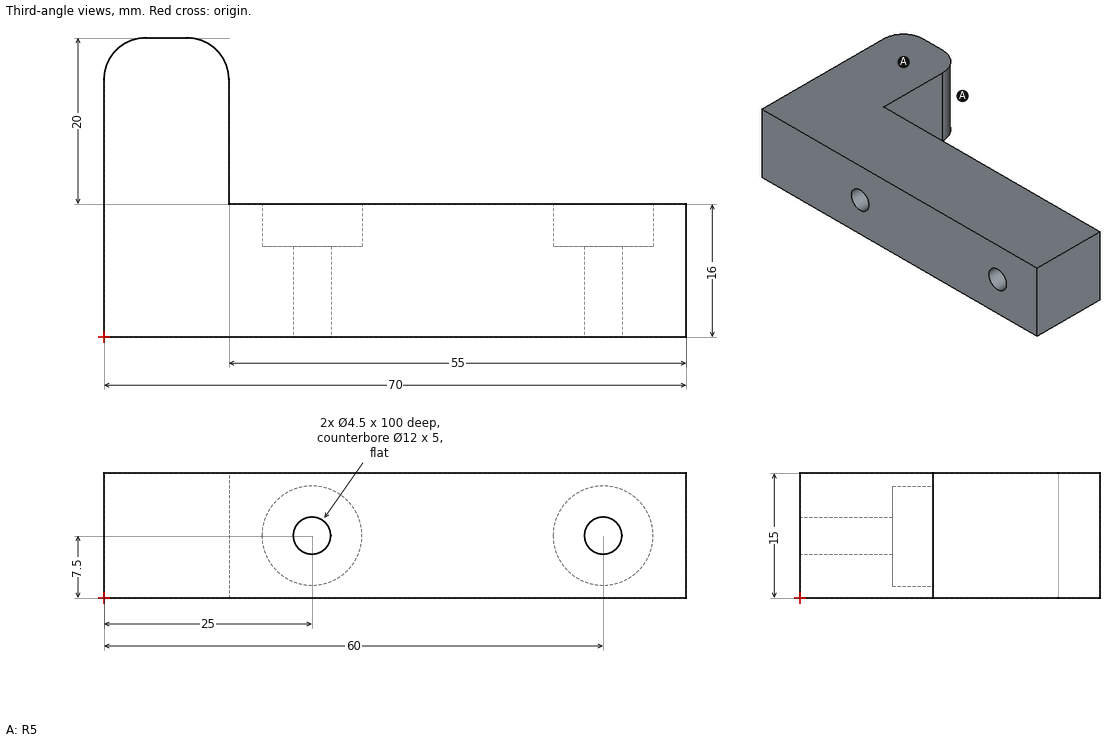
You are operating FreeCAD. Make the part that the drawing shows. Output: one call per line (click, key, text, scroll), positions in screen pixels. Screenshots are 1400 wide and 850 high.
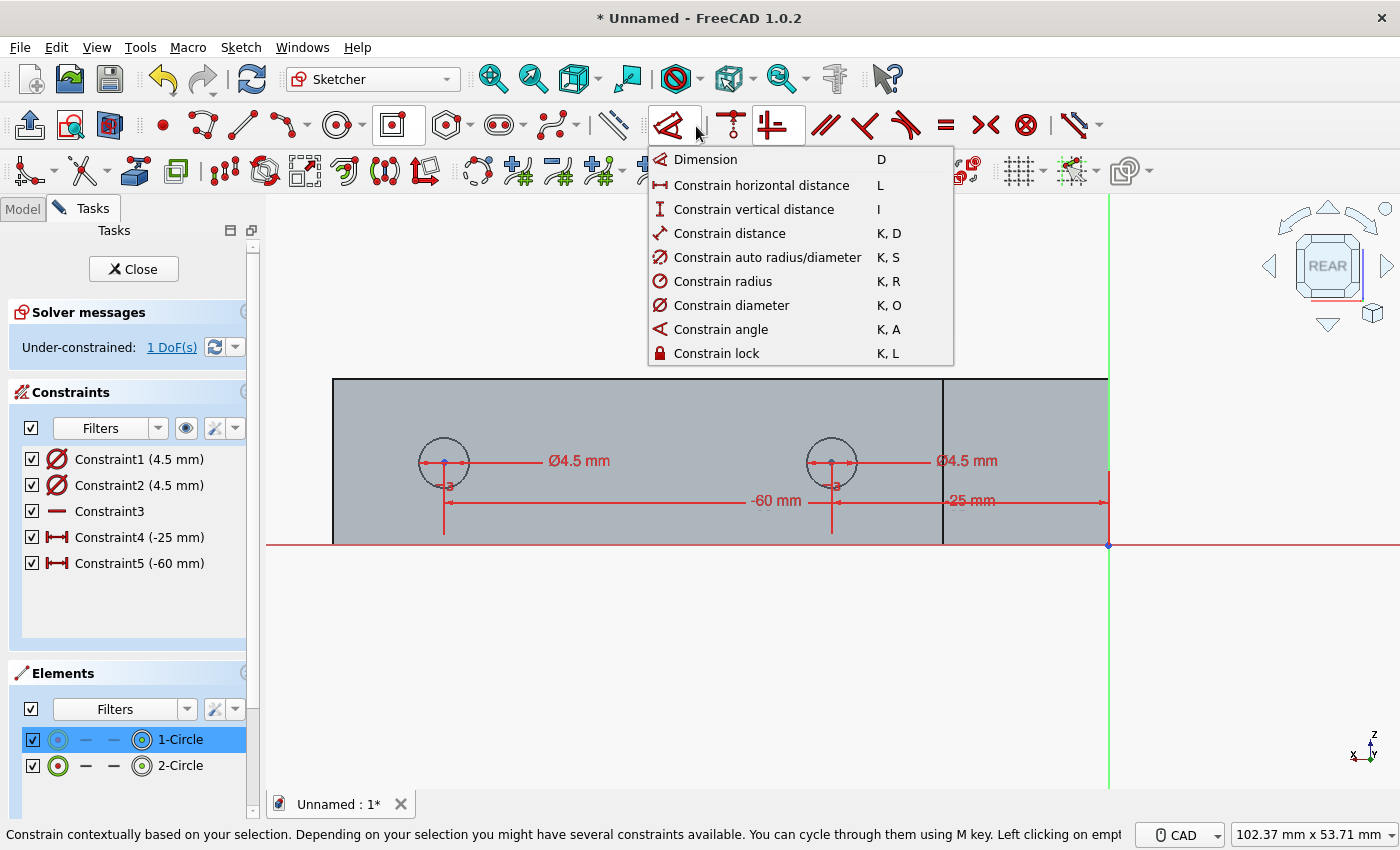
click(801, 209)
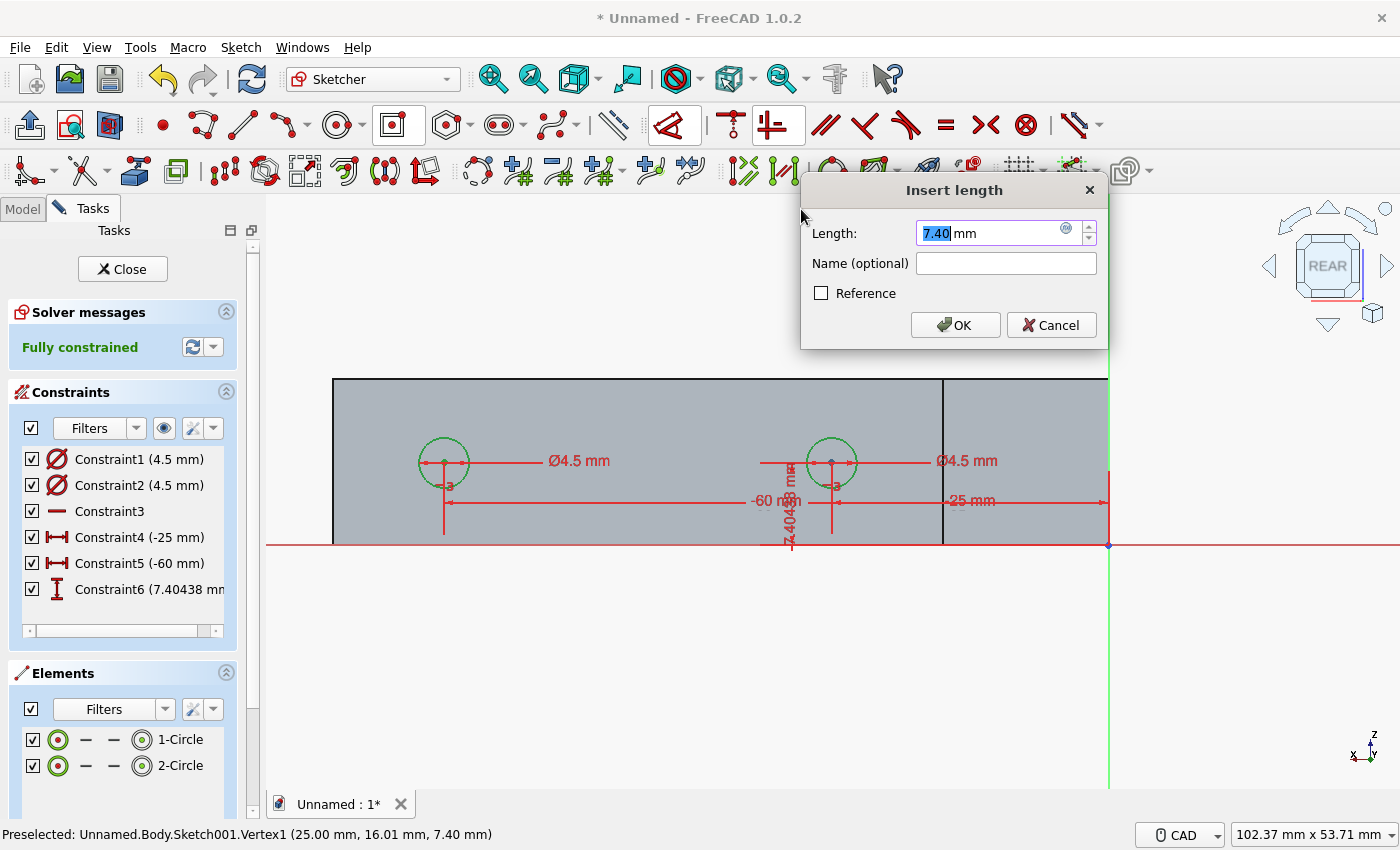
text(7.5)
key(Return)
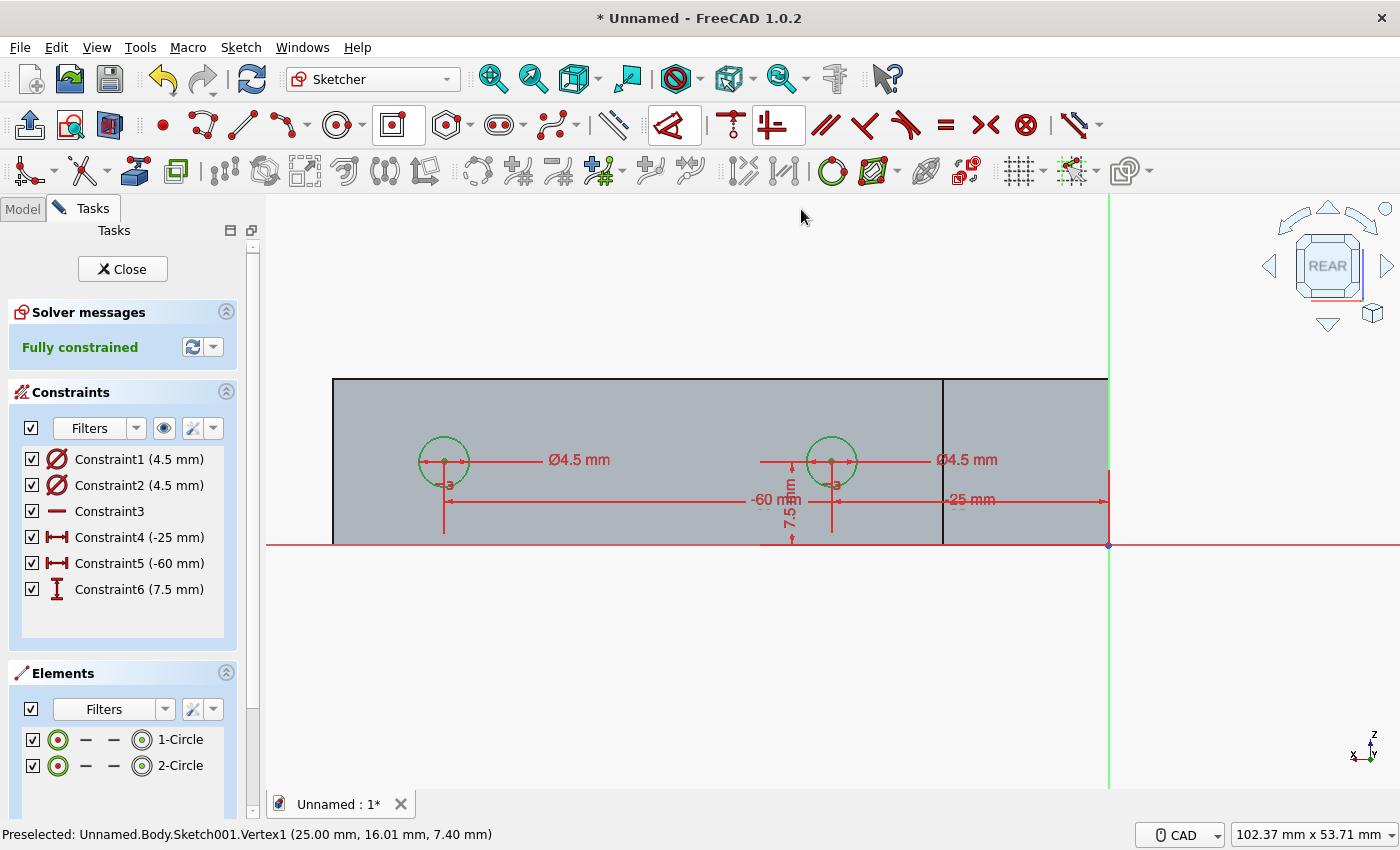
click(123, 269)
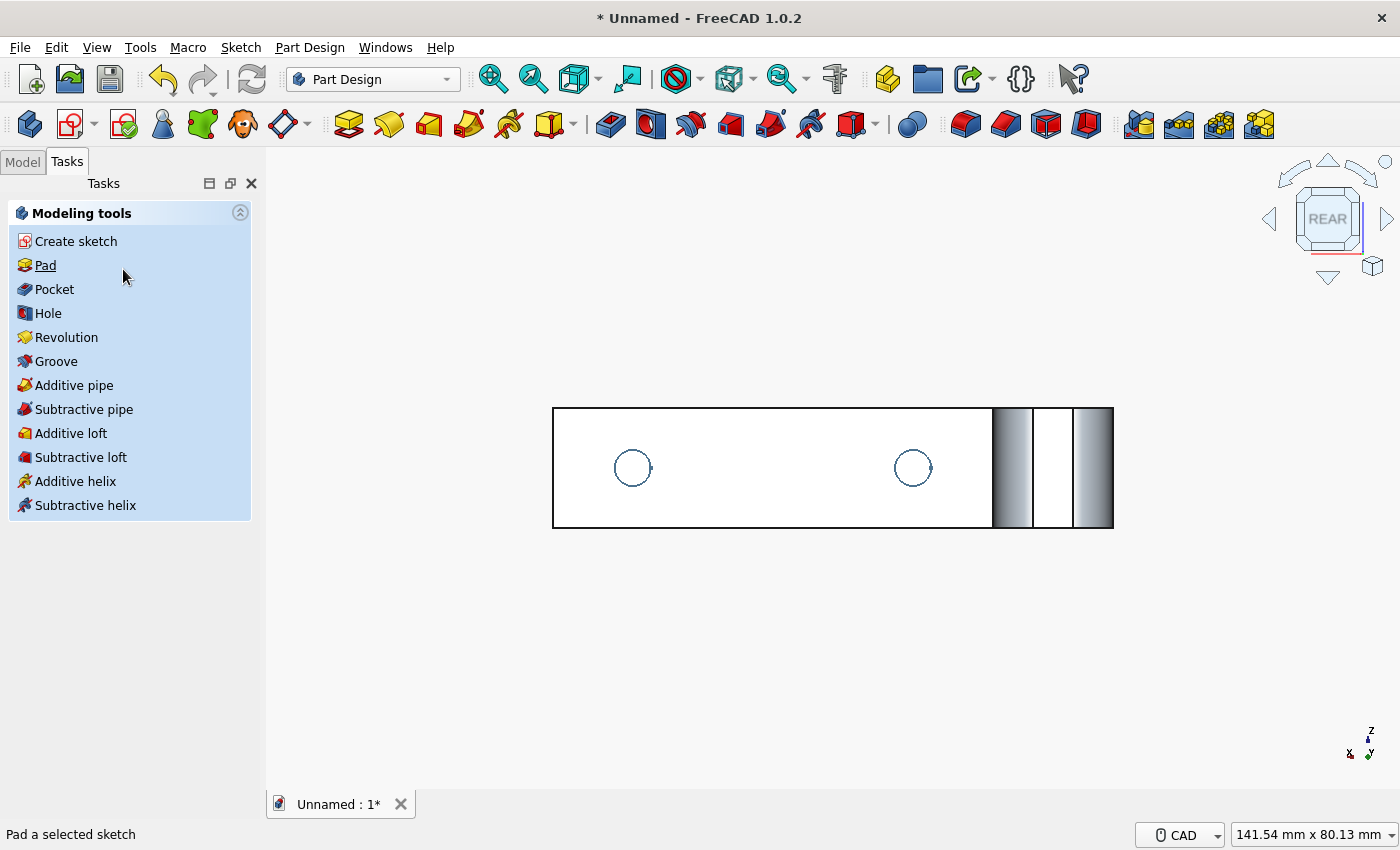
click(652, 124)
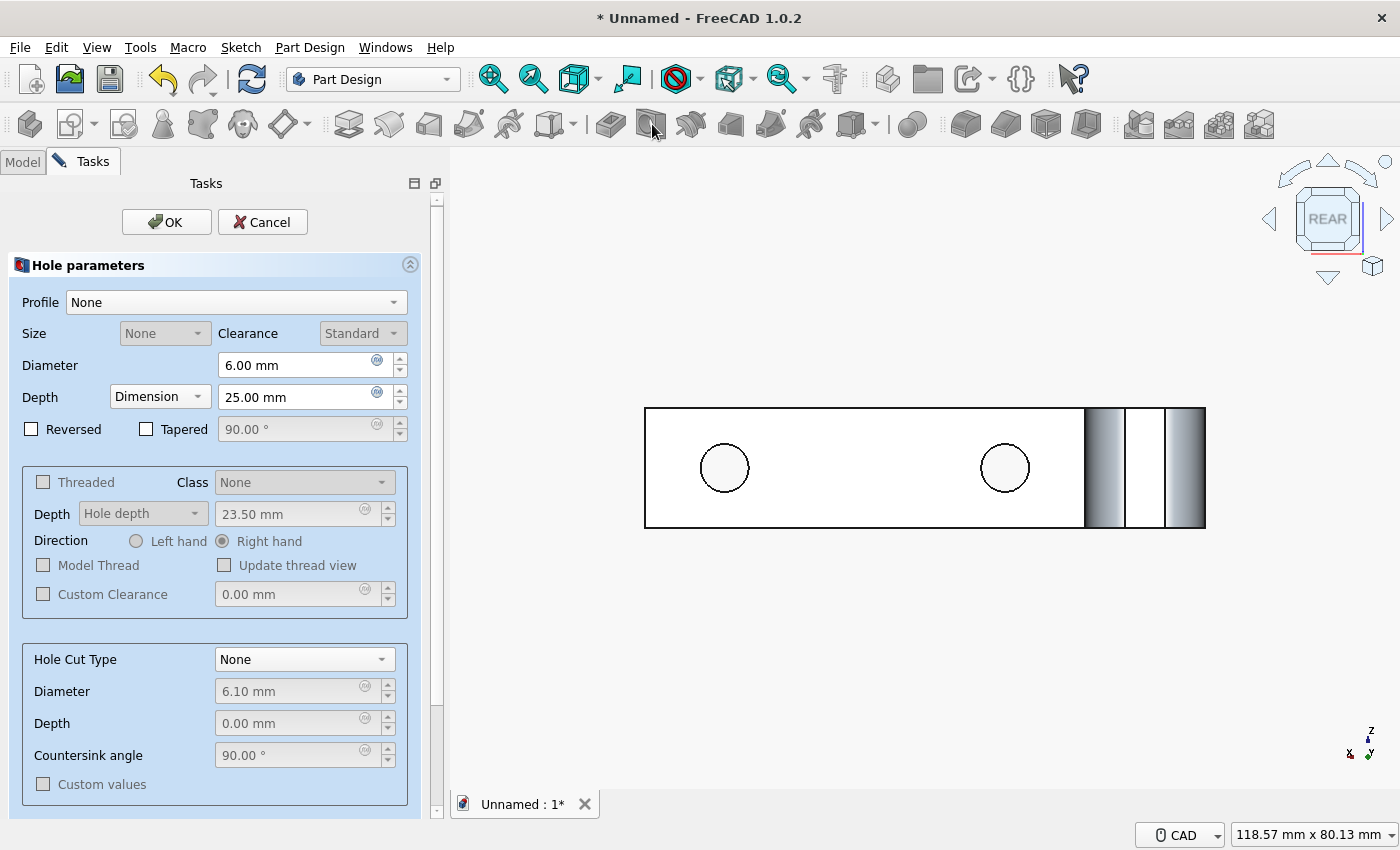
triple_click(305, 365)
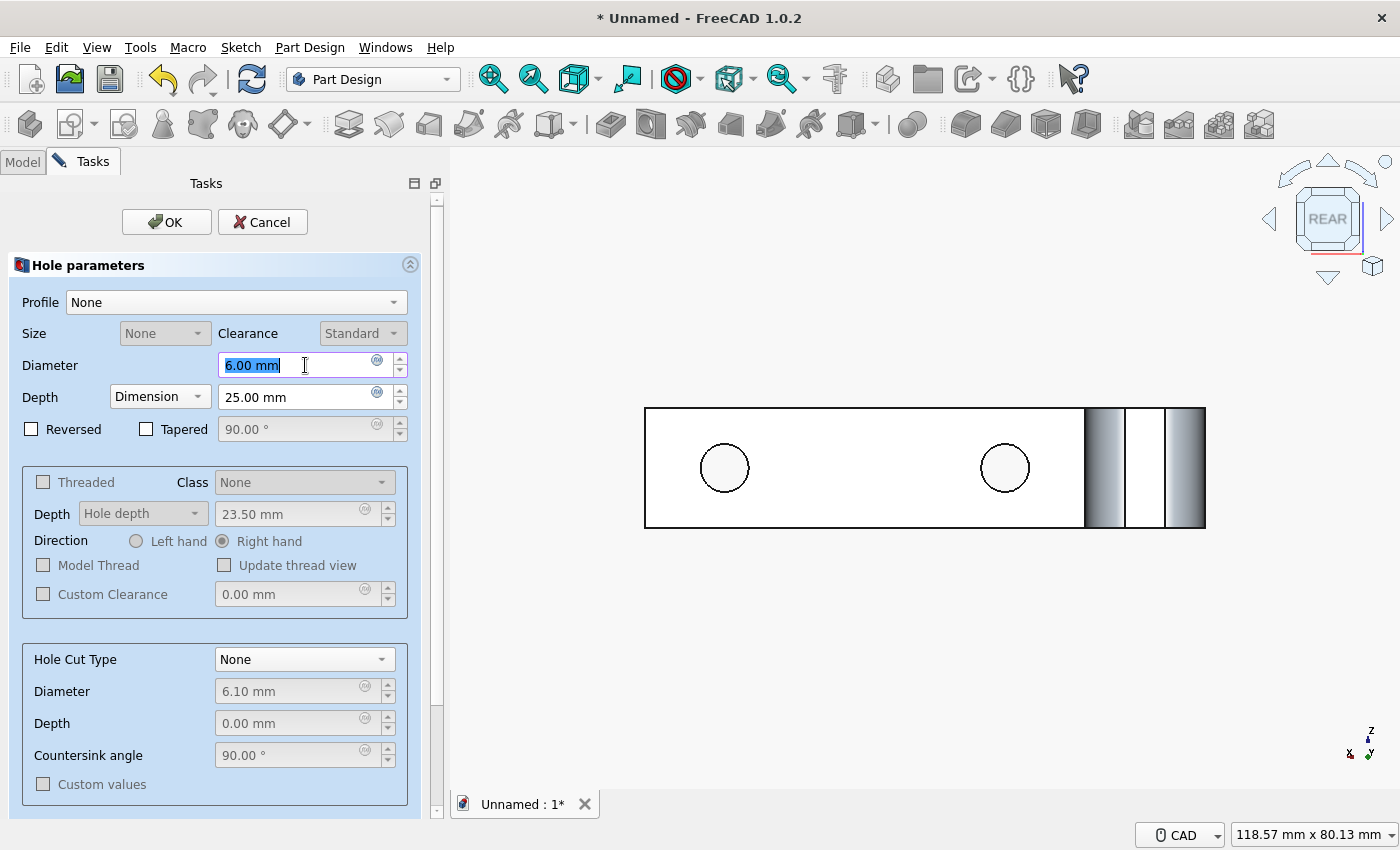
text(4.5)
key(Tab)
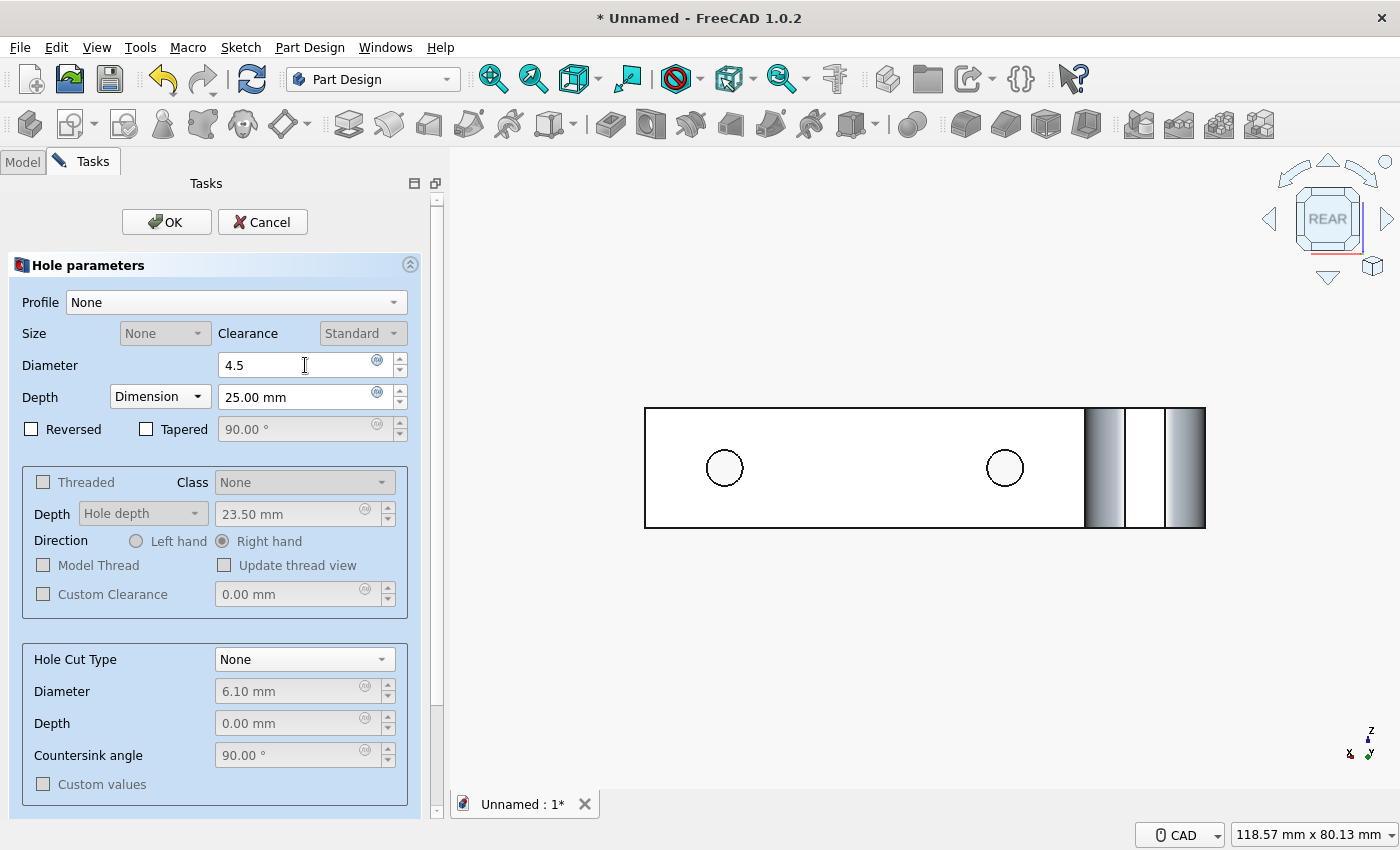
triple_click(305, 397)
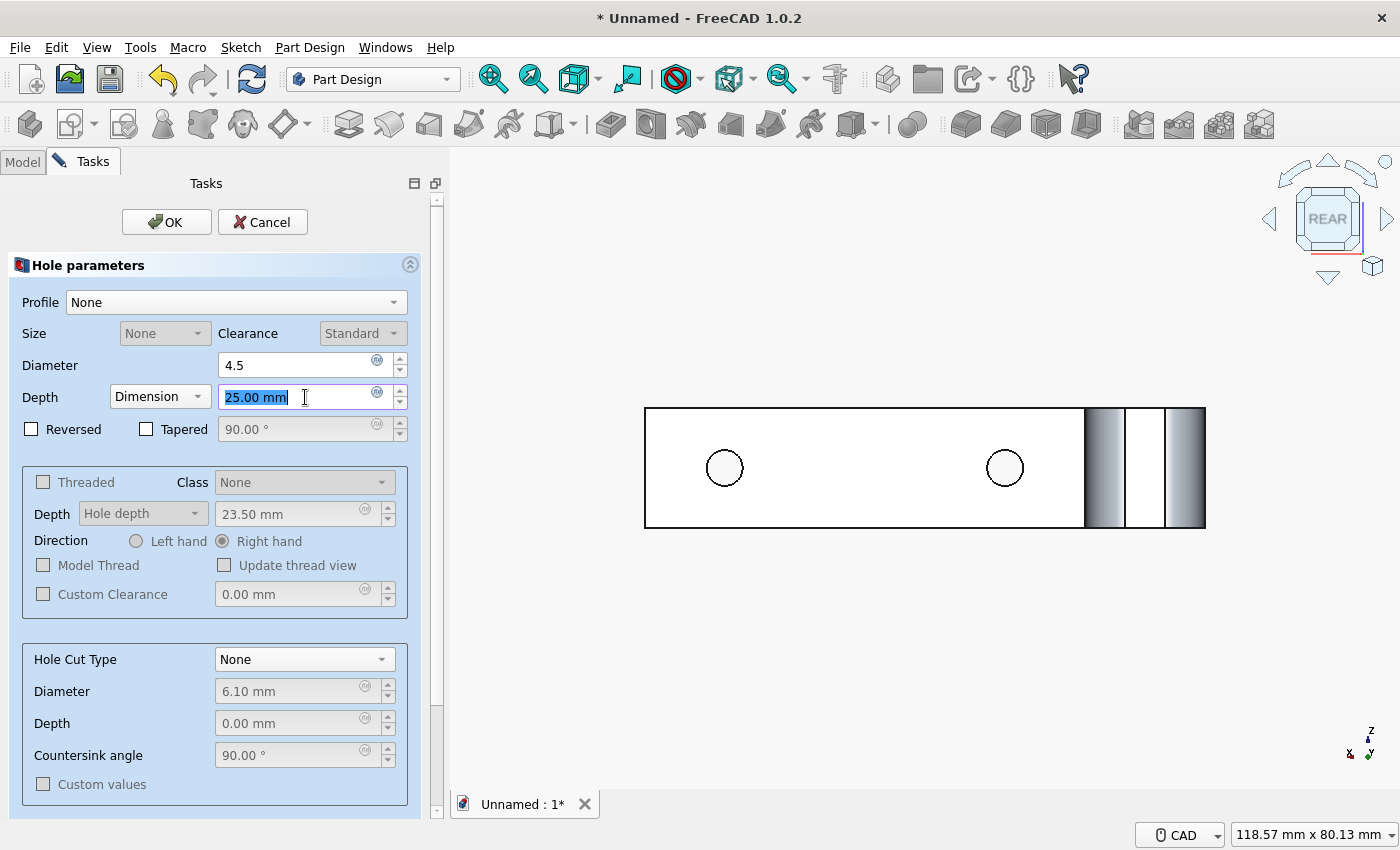
text(100)
key(Tab)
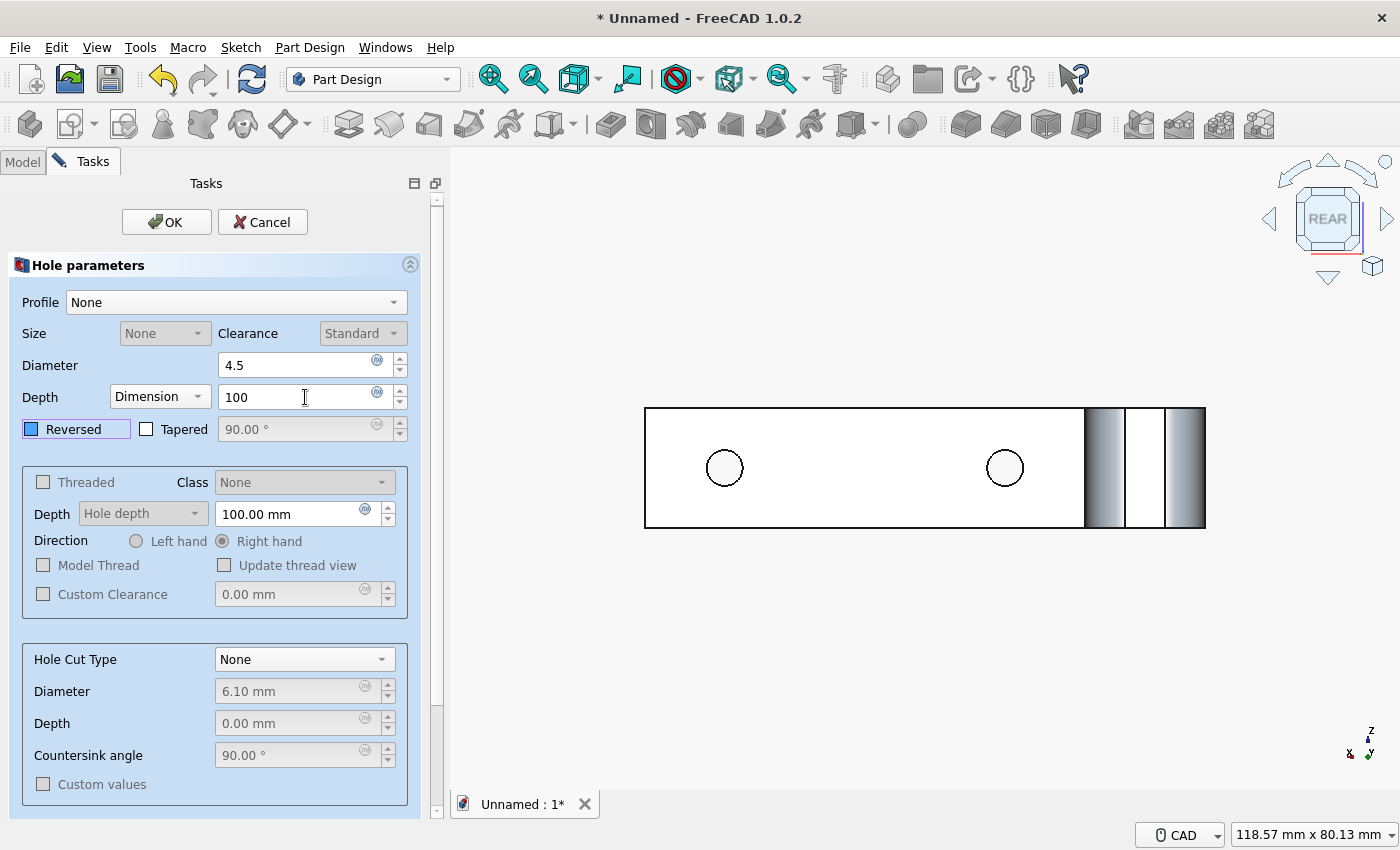
click(306, 660)